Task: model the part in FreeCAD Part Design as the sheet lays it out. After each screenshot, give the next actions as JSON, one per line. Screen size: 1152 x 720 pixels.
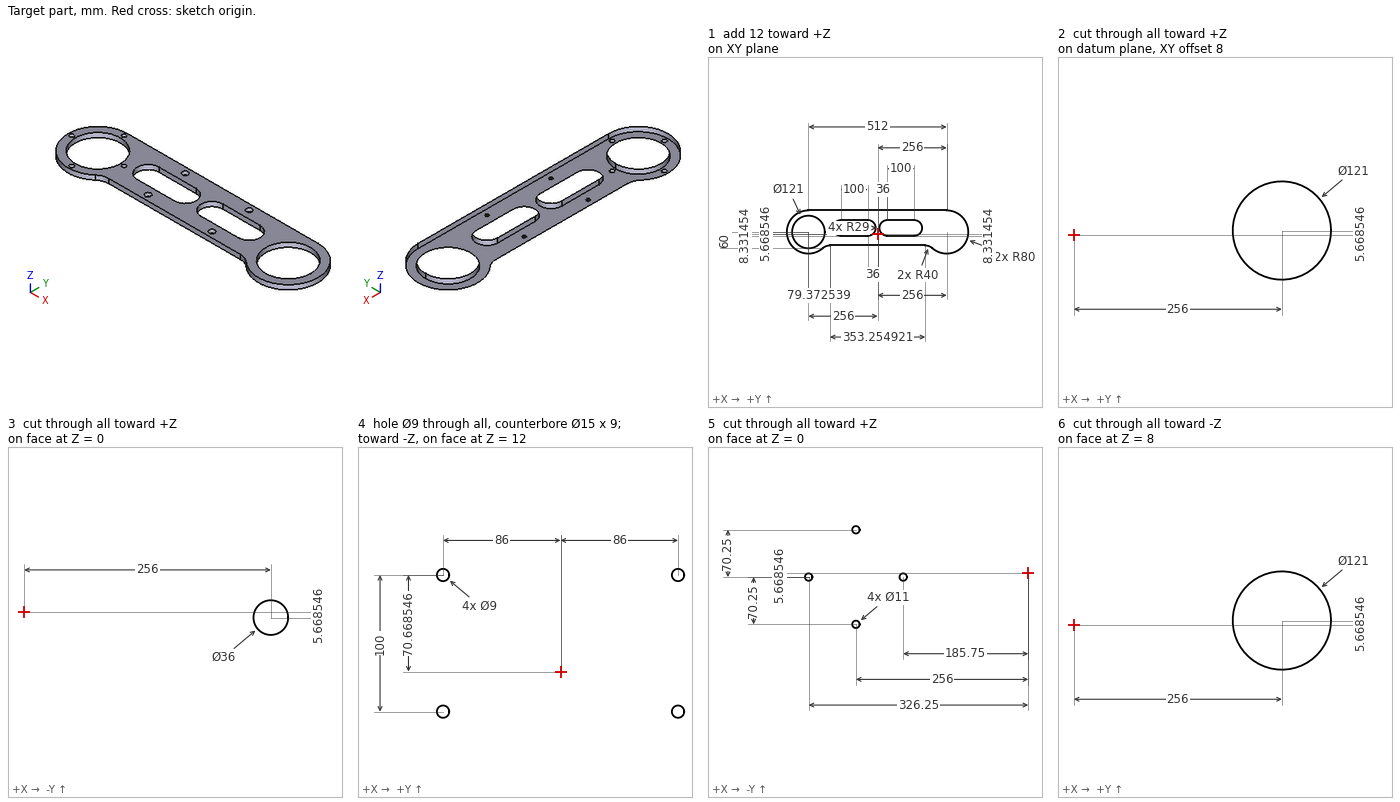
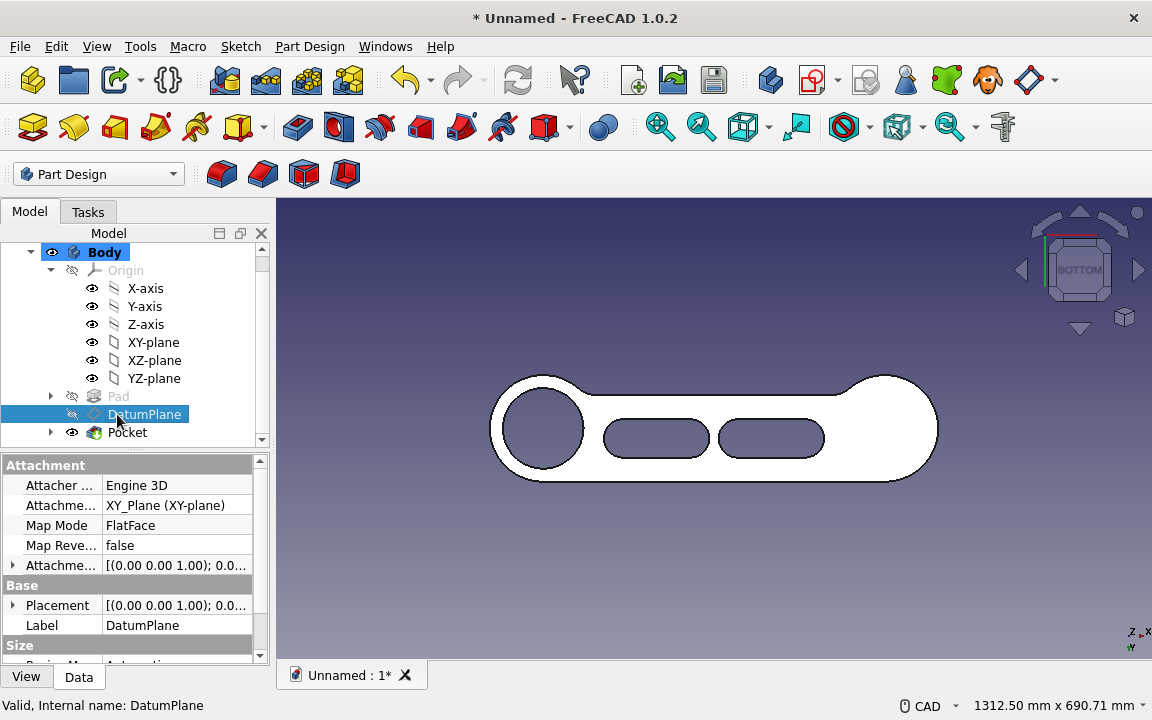
{"action": "left_click", "coordinate": [906, 427]}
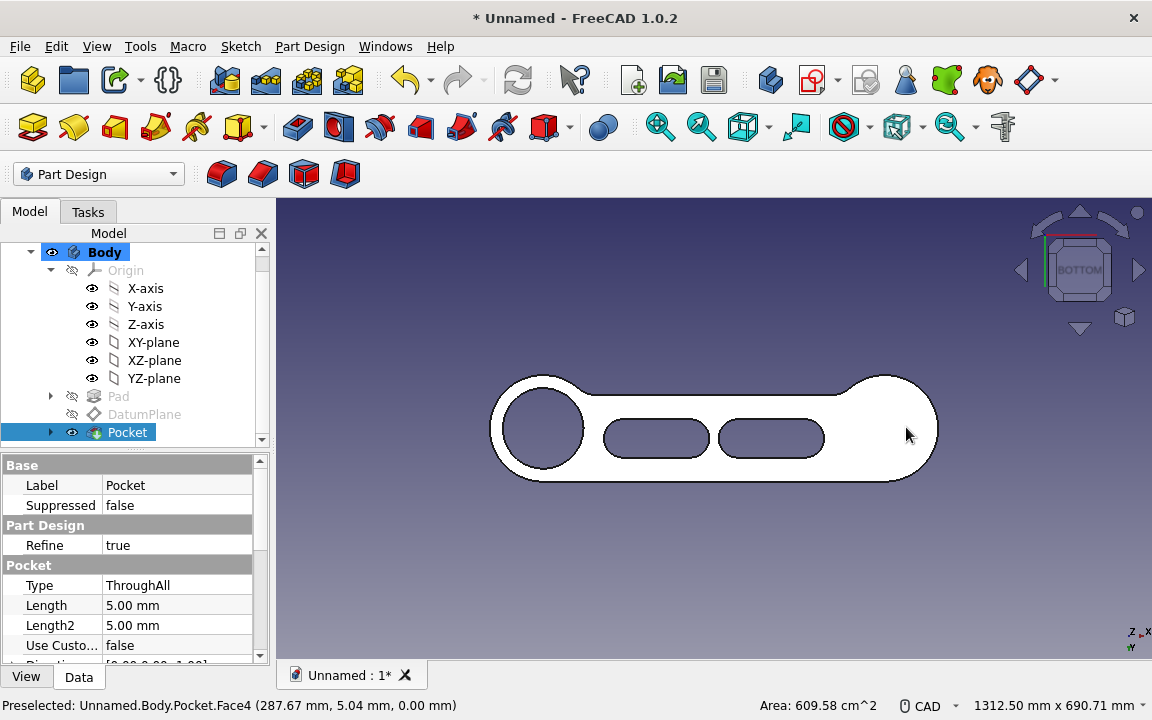
{"action": "left_click", "coordinate": [812, 80]}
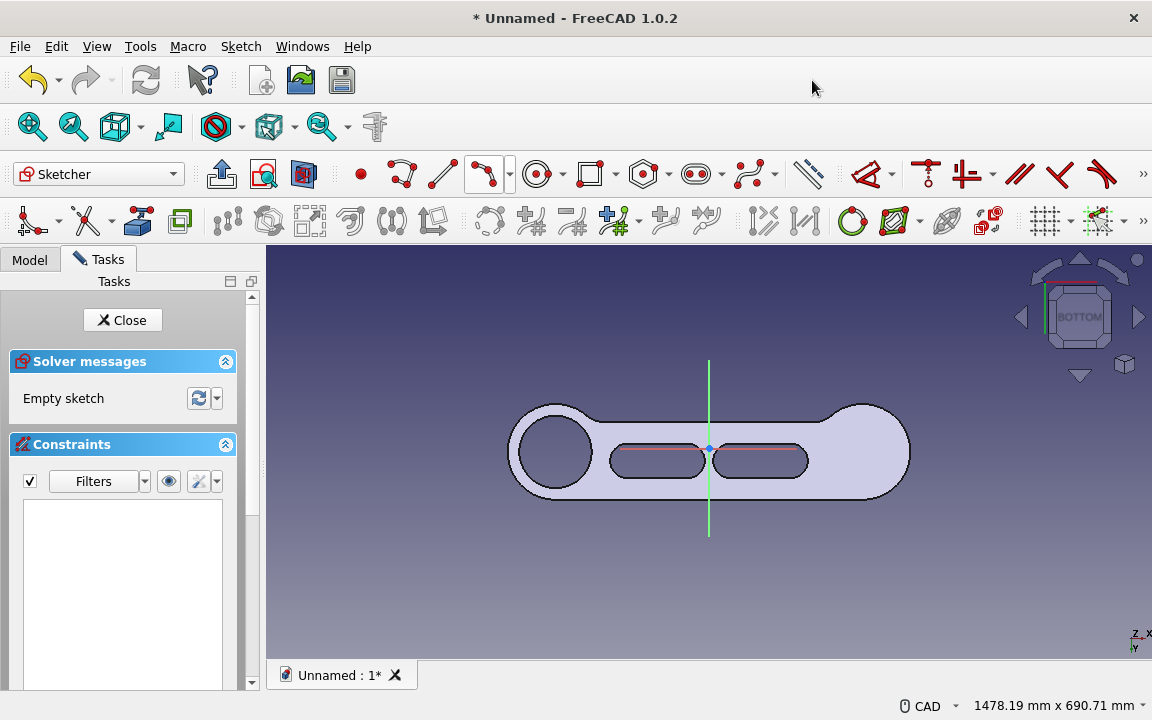
{"action": "scroll", "coordinate": [885, 452], "scroll_direction": "up", "scroll_amount": 12}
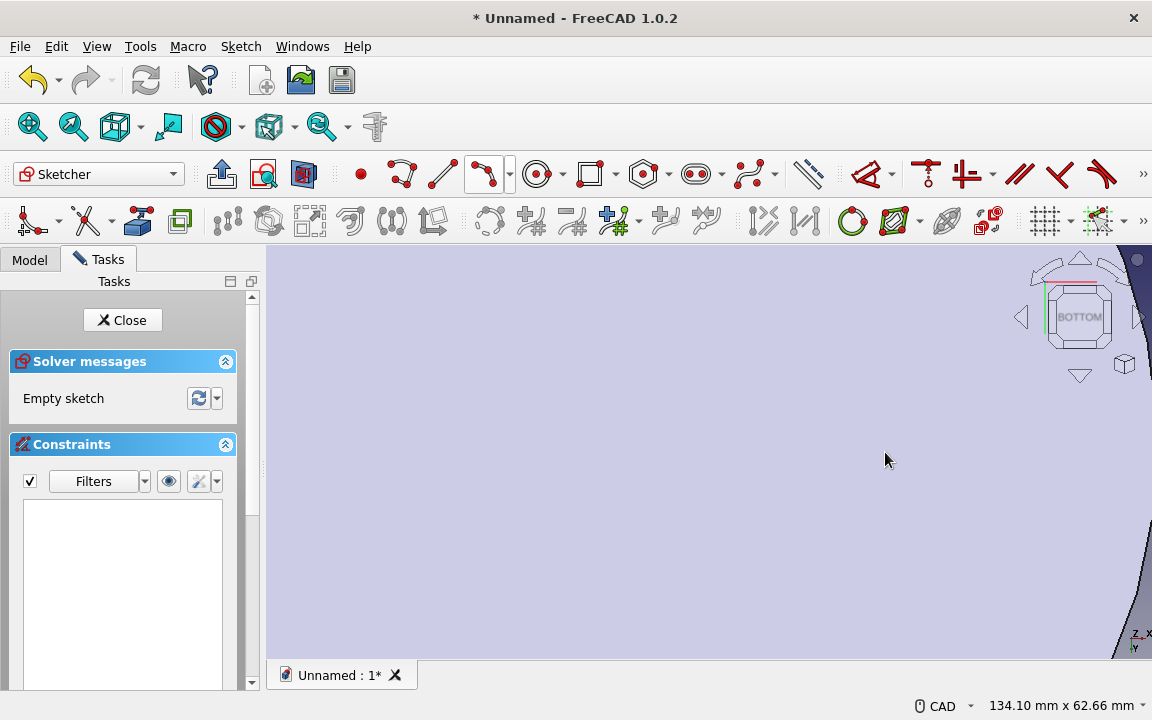
{"action": "left_click", "coordinate": [536, 174]}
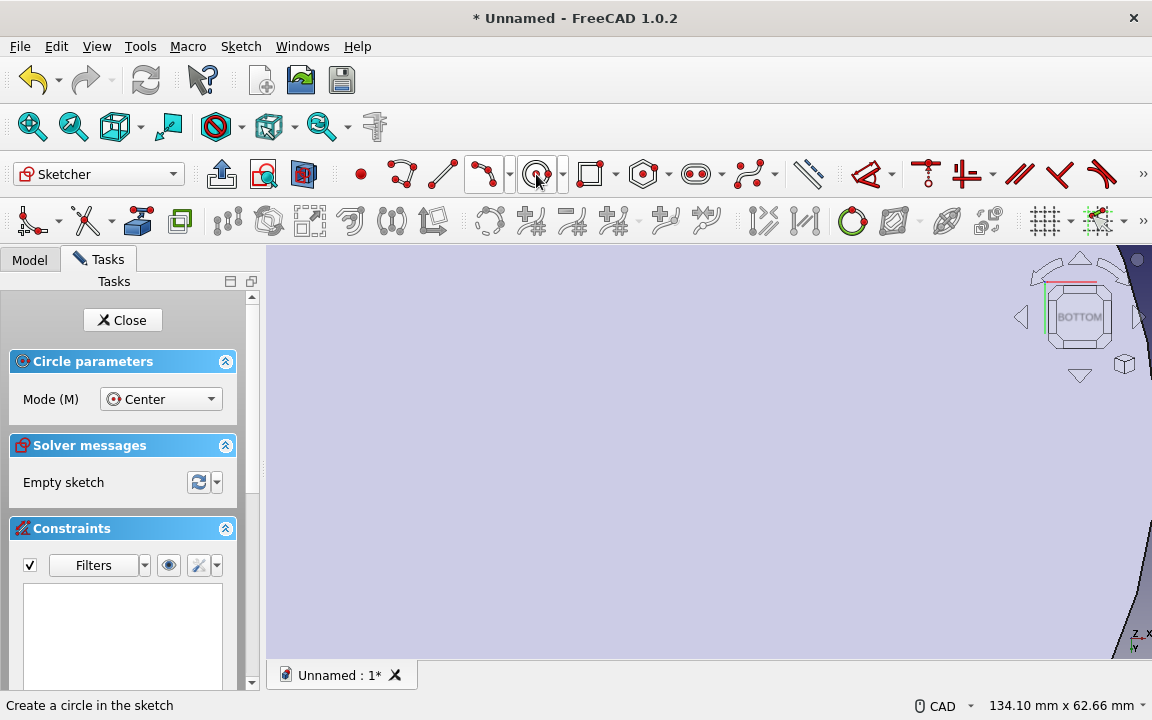
{"action": "left_click", "coordinate": [629, 446]}
{"action": "mouse_move", "coordinate": [713, 362]}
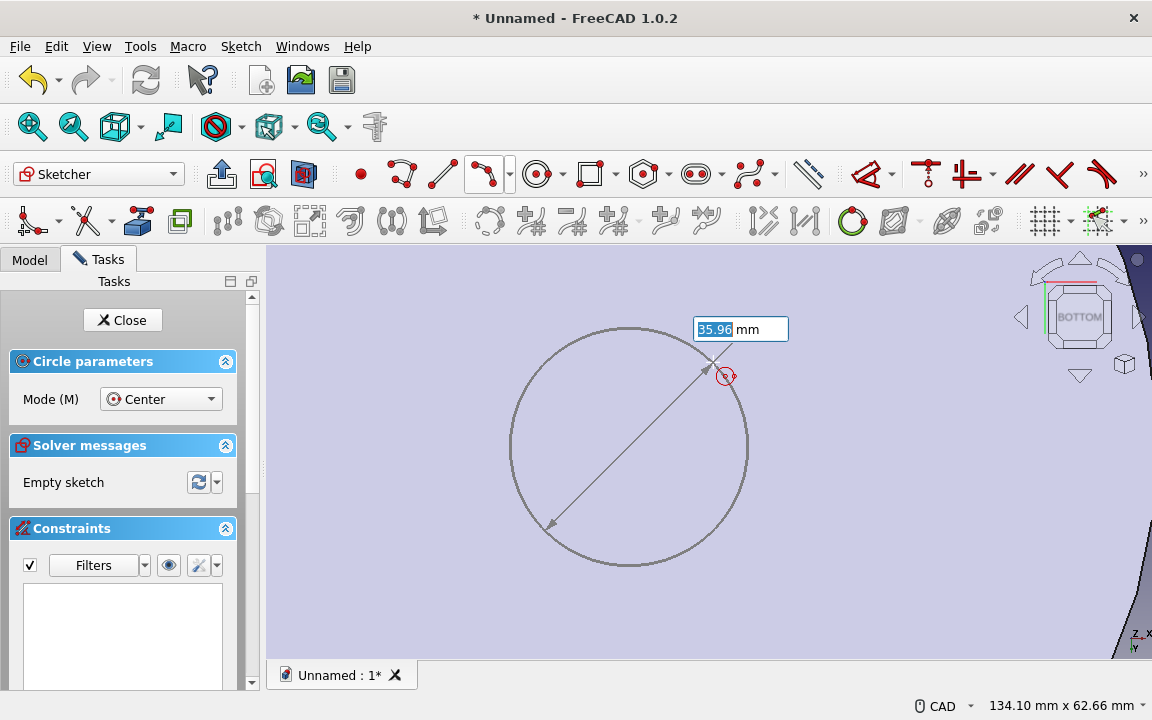
{"action": "type", "text": "36"}
{"action": "key", "text": "Return"}
{"action": "key", "text": "Escape"}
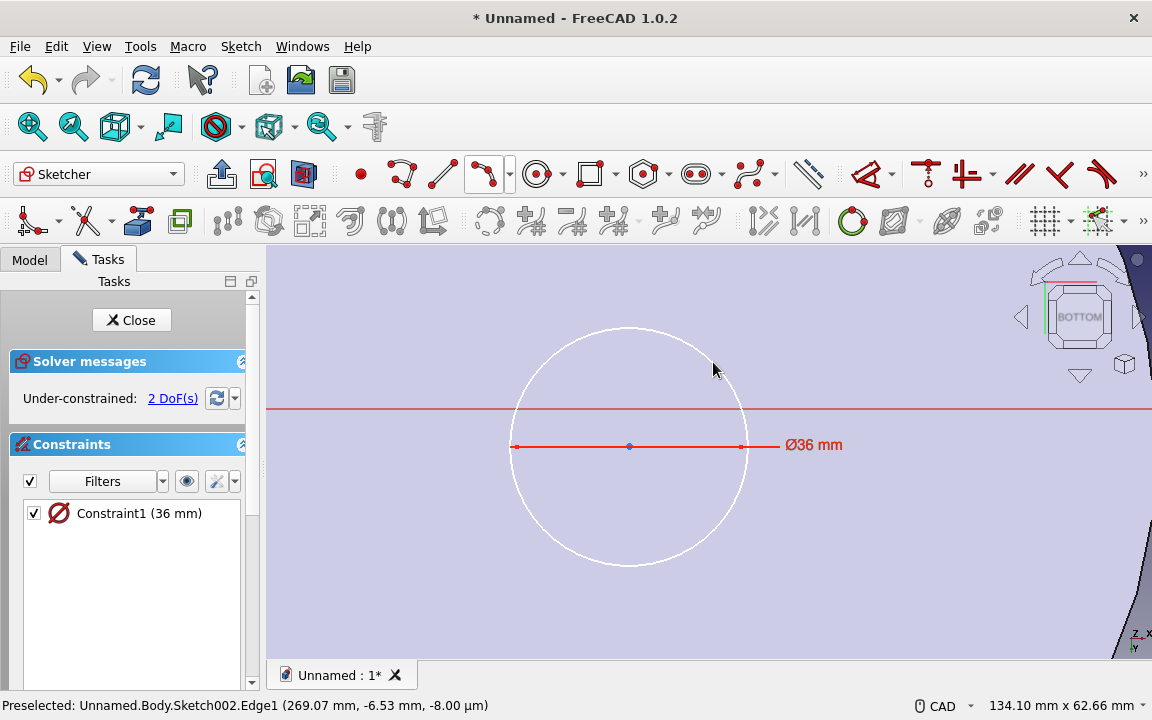
{"action": "left_click", "coordinate": [866, 174]}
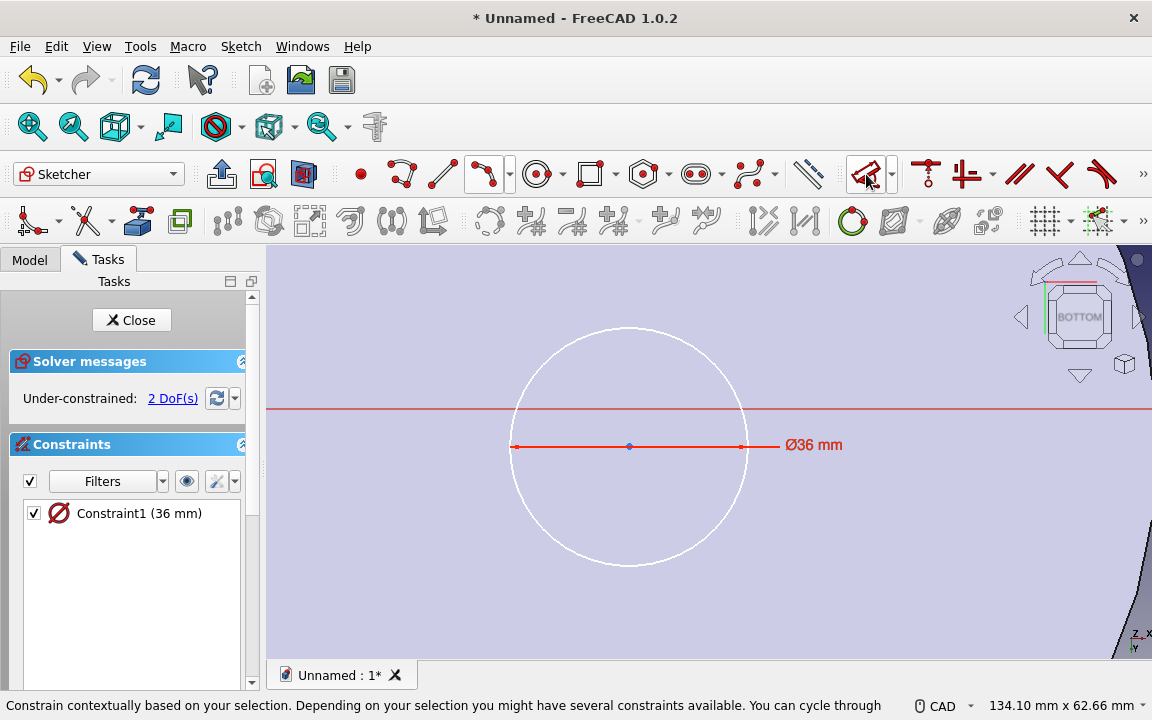
{"action": "left_click", "coordinate": [629, 447]}
{"action": "left_click", "coordinate": [462, 375]}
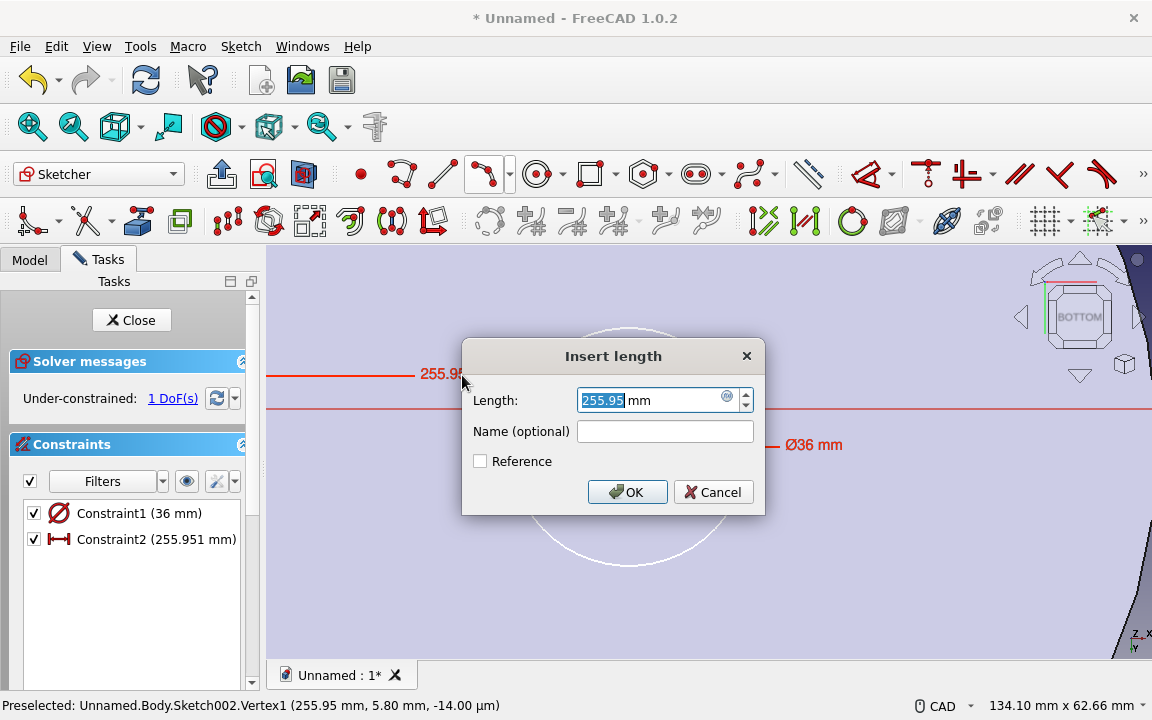
{"action": "type", "text": "256"}
{"action": "key", "text": "Return"}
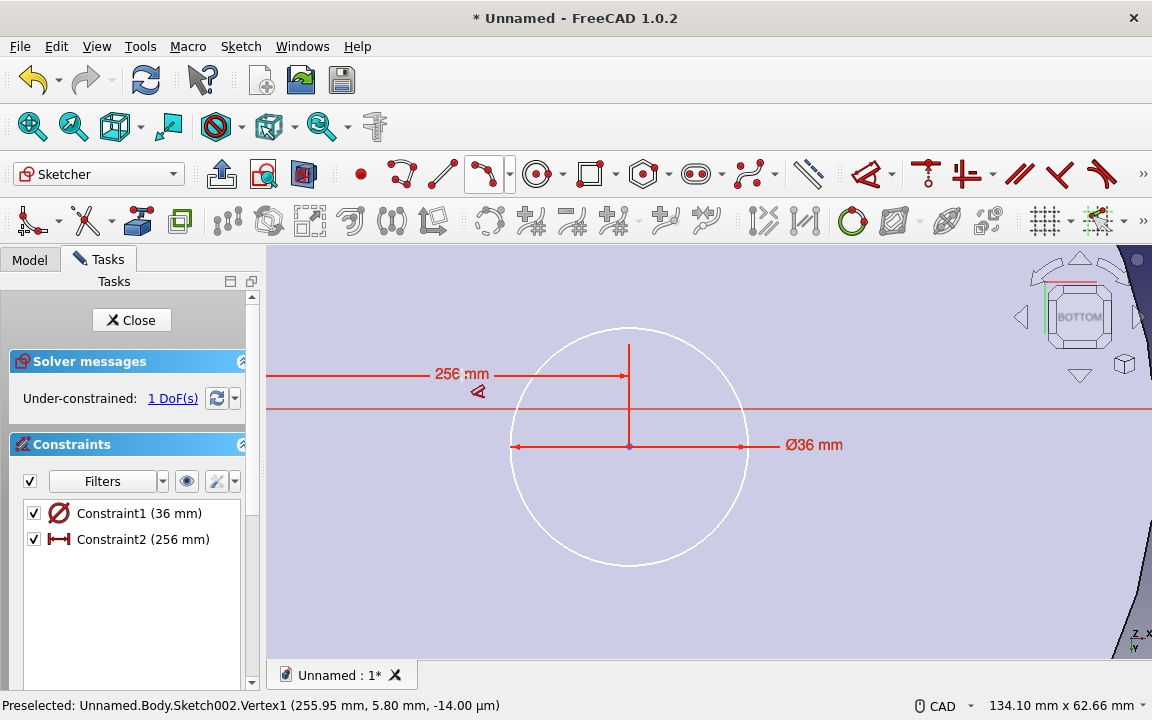
{"action": "left_click", "coordinate": [629, 447]}
{"action": "left_click", "coordinate": [663, 428]}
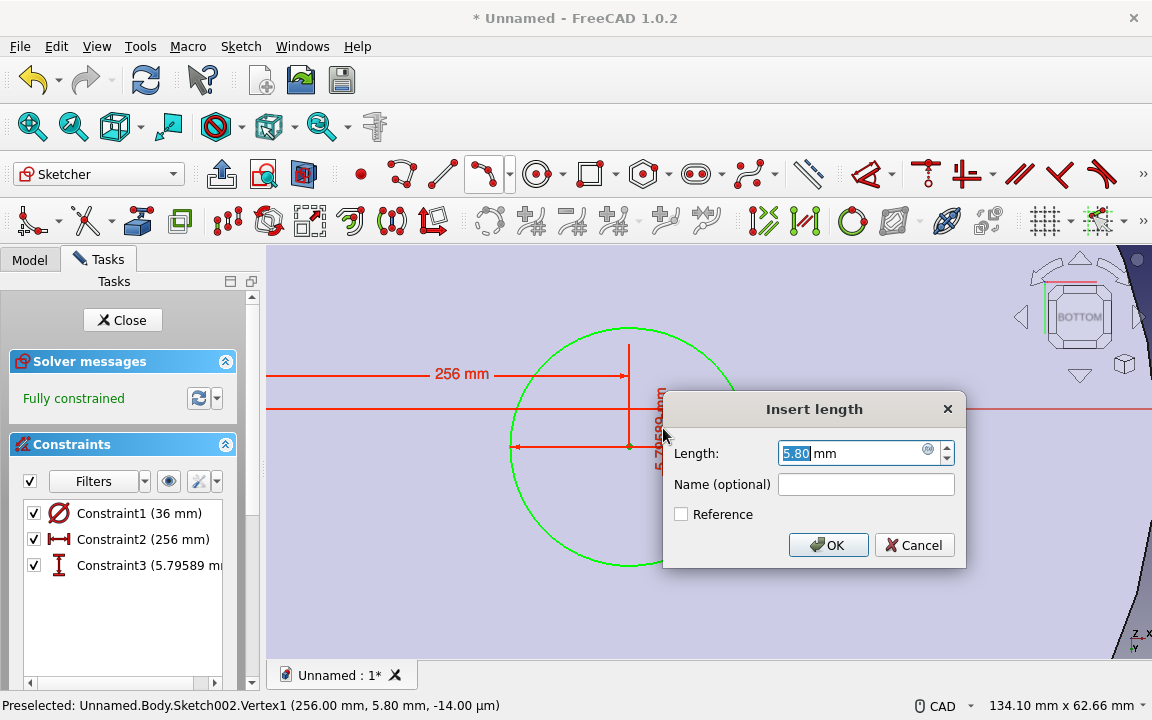
{"action": "type", "text": "5.668546"}
{"action": "key", "text": "Return"}
{"action": "key", "text": "Escape"}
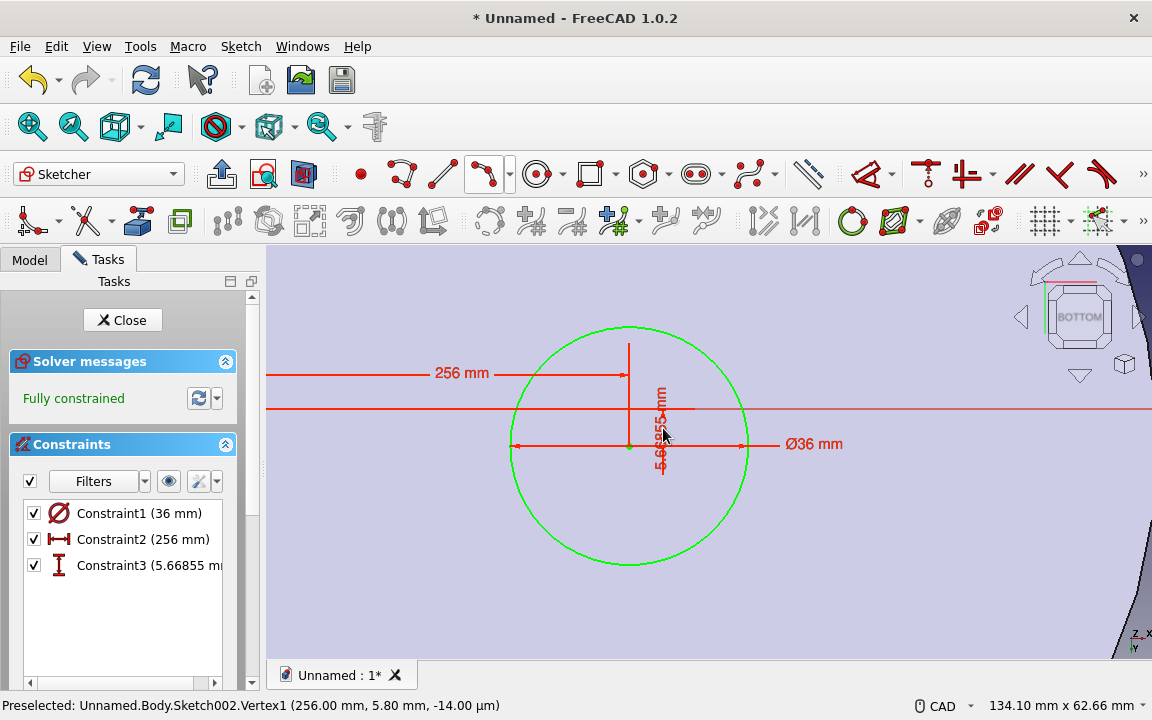
{"action": "left_click", "coordinate": [123, 320]}